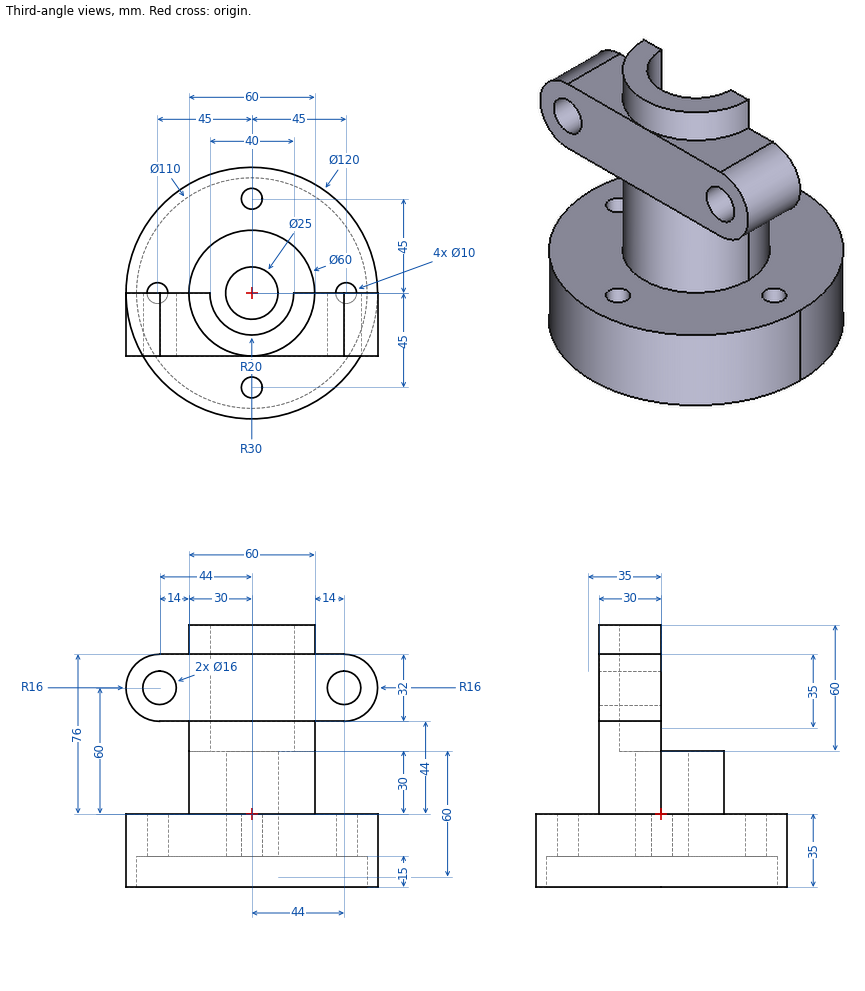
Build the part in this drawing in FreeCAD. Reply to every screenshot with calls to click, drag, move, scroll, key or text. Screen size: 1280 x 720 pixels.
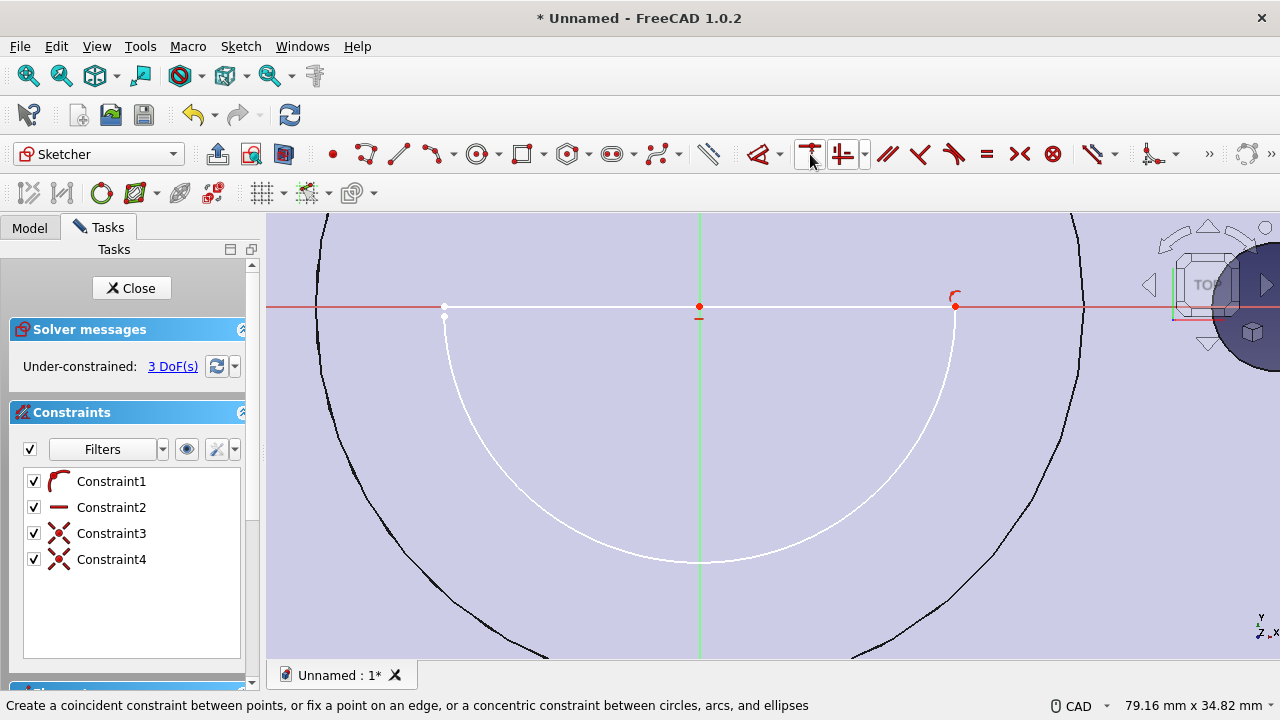
click(758, 154)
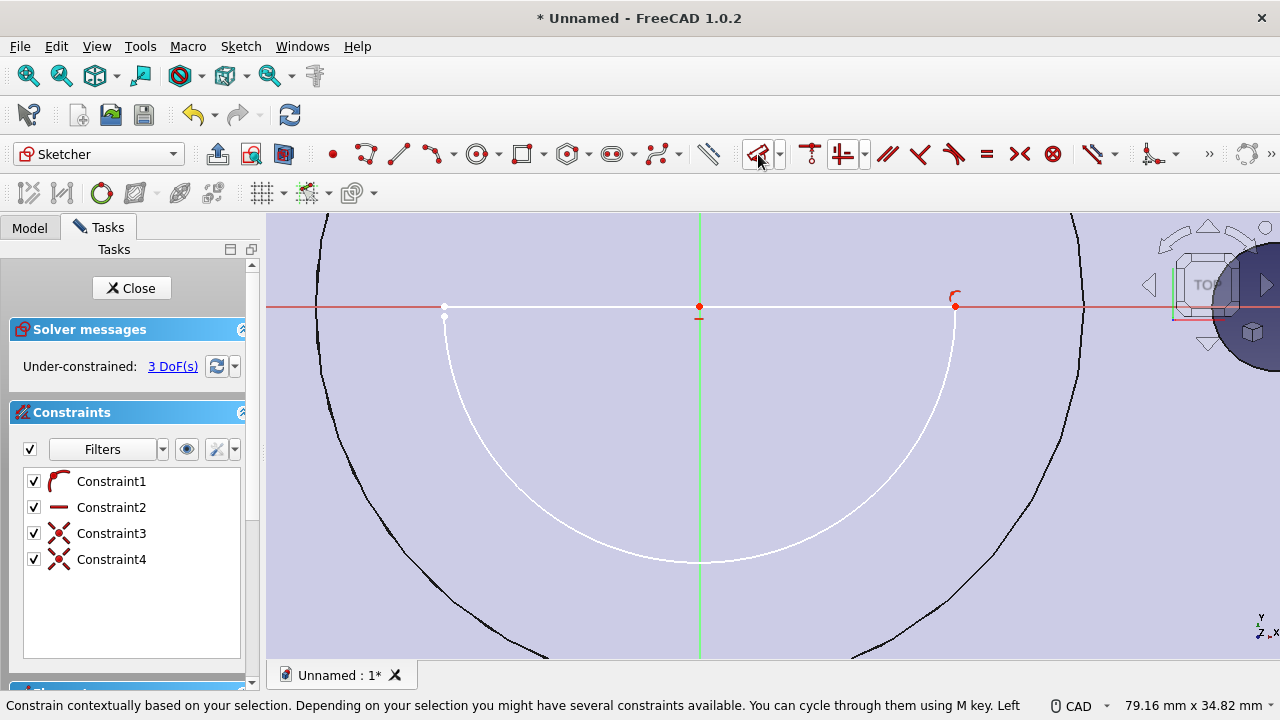
click(555, 518)
click(537, 544)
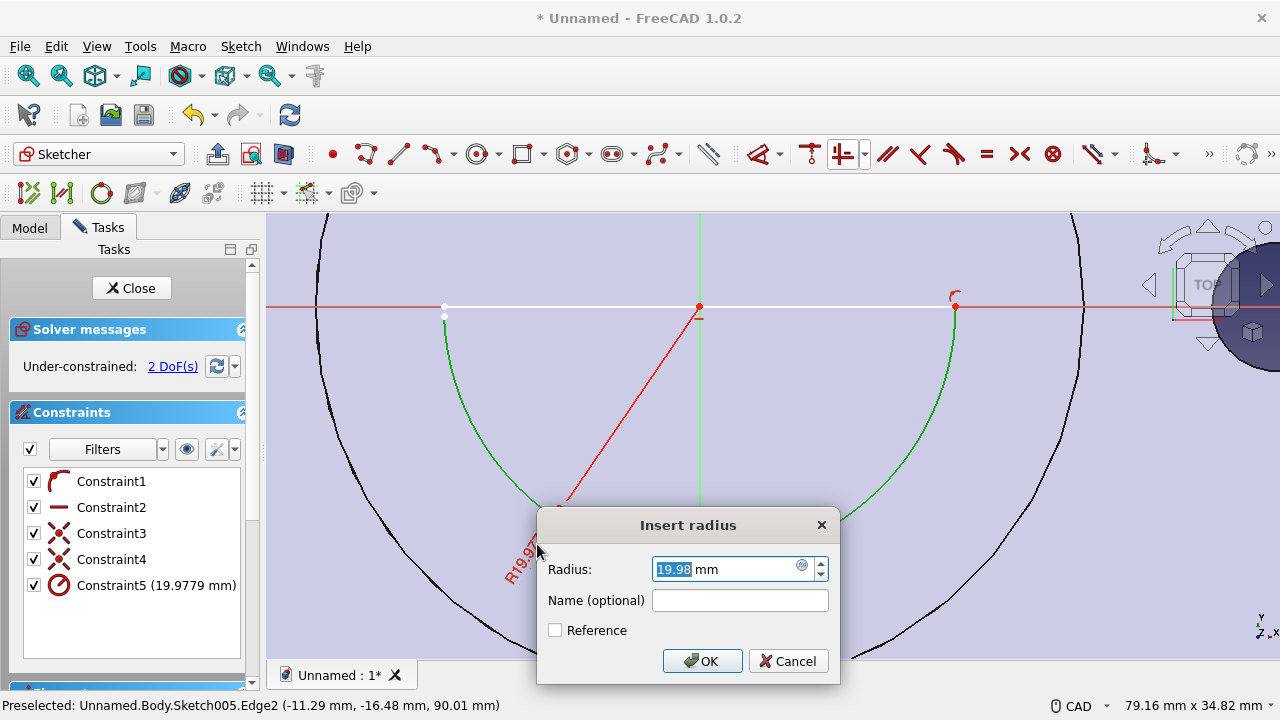
text(20)
key(Return)
key(Escape)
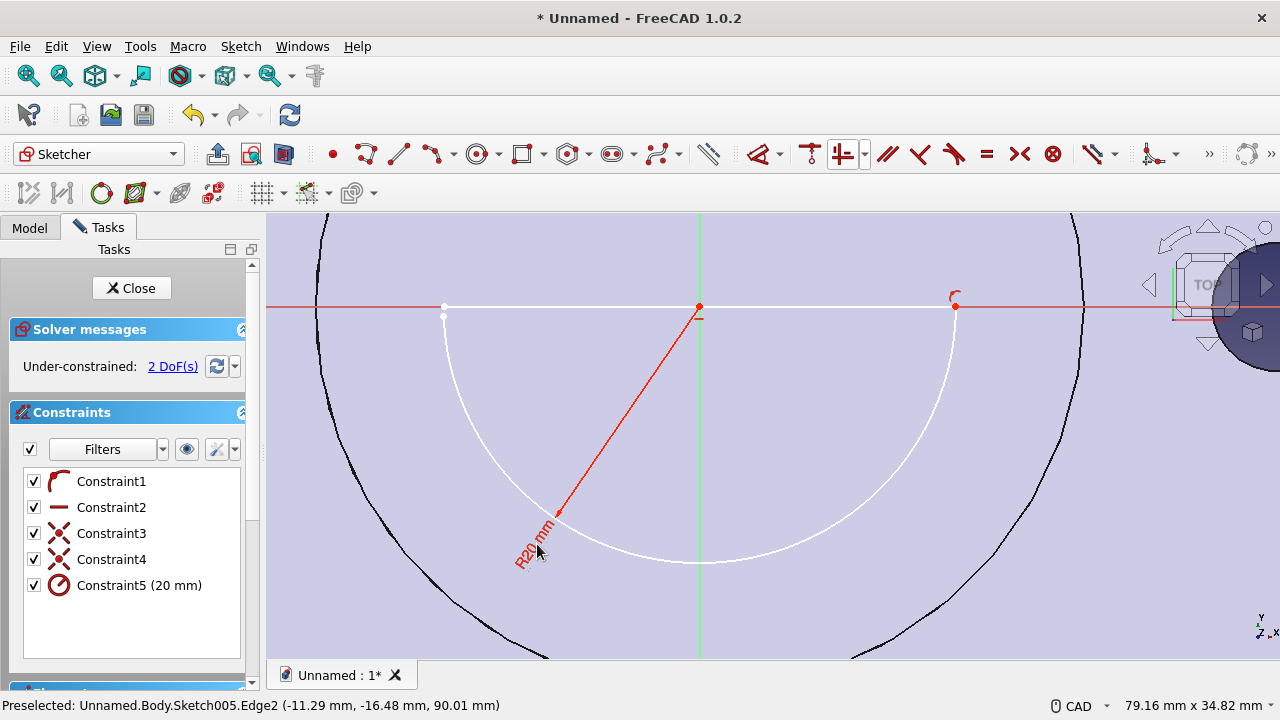
click(444, 317)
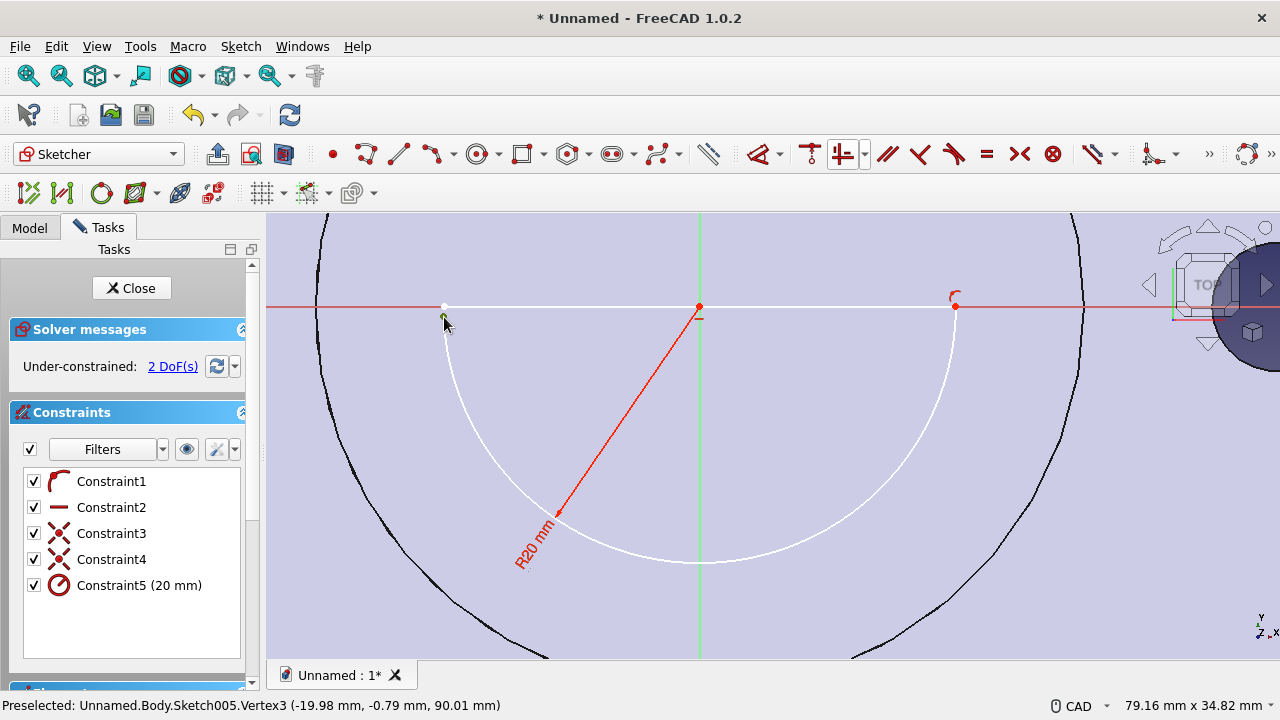
click(353, 307)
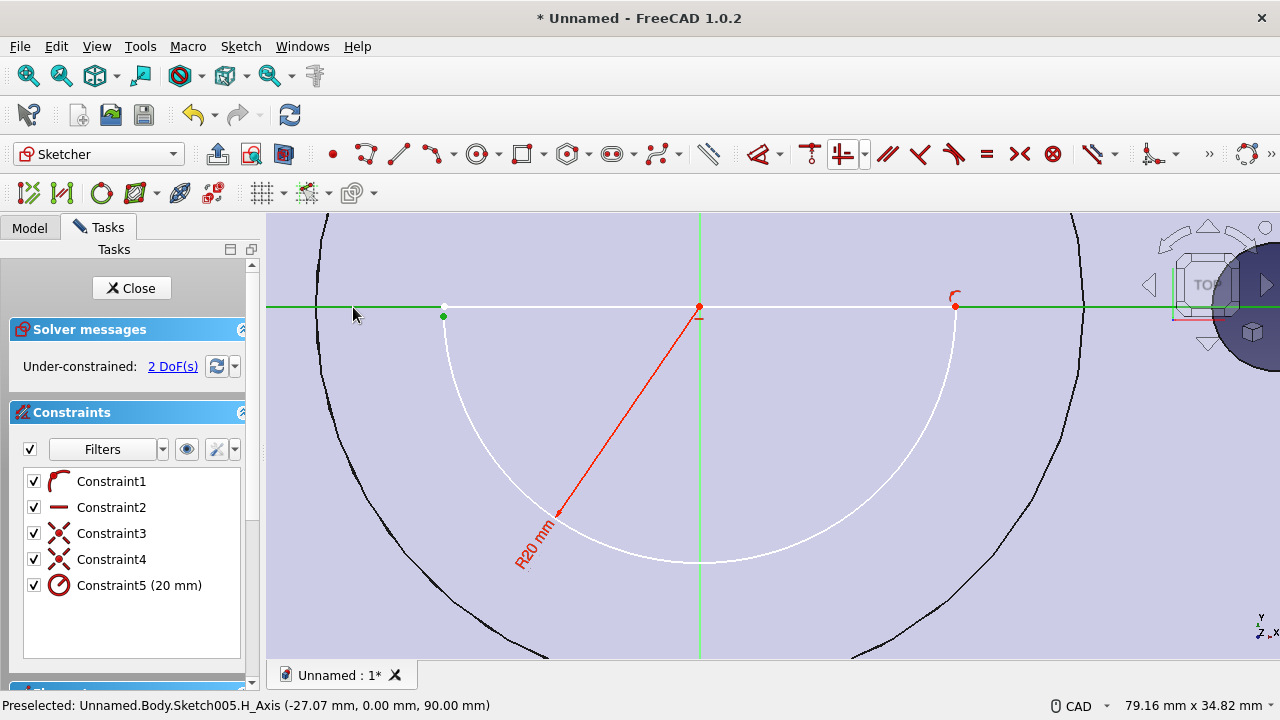
click(810, 154)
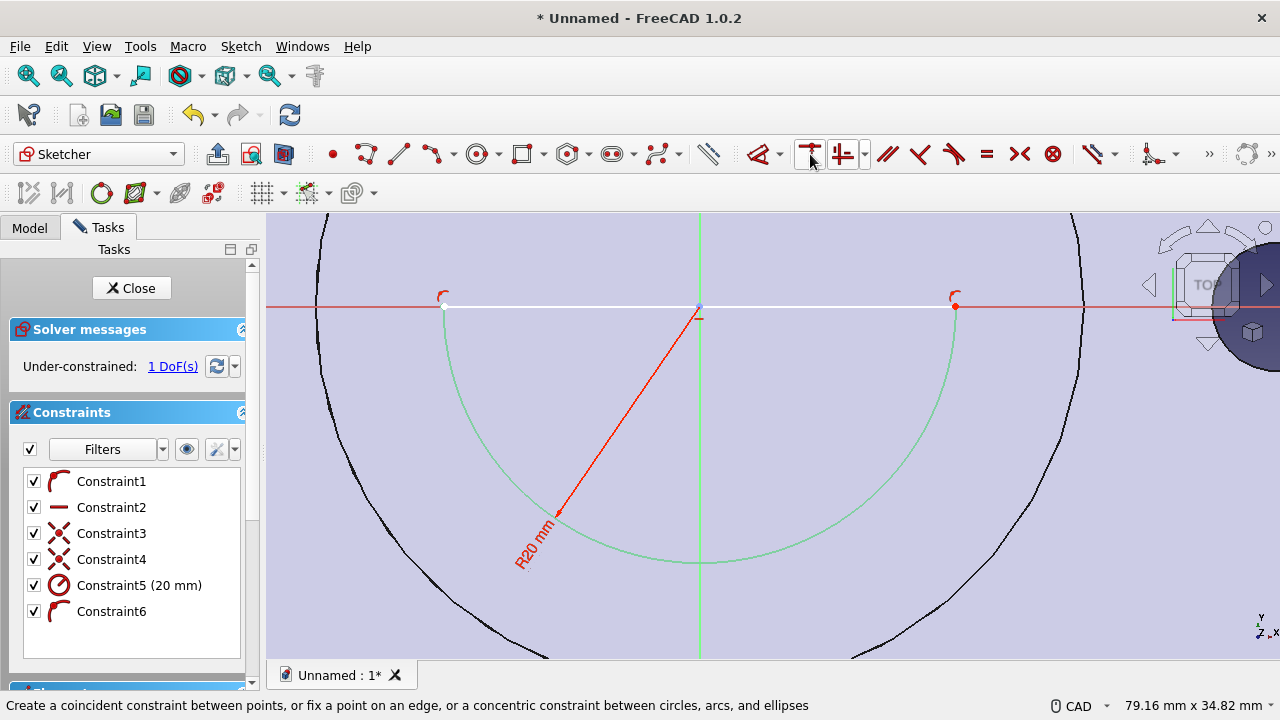
click(758, 154)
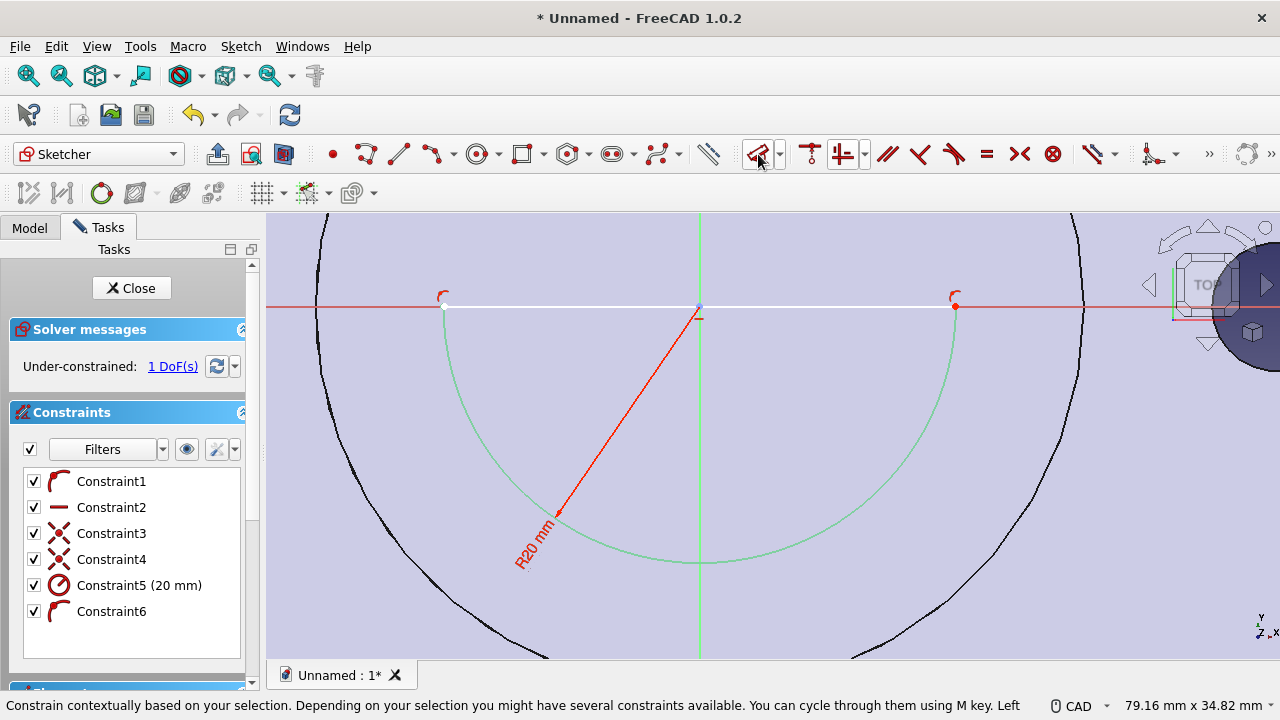
click(802, 307)
click(582, 273)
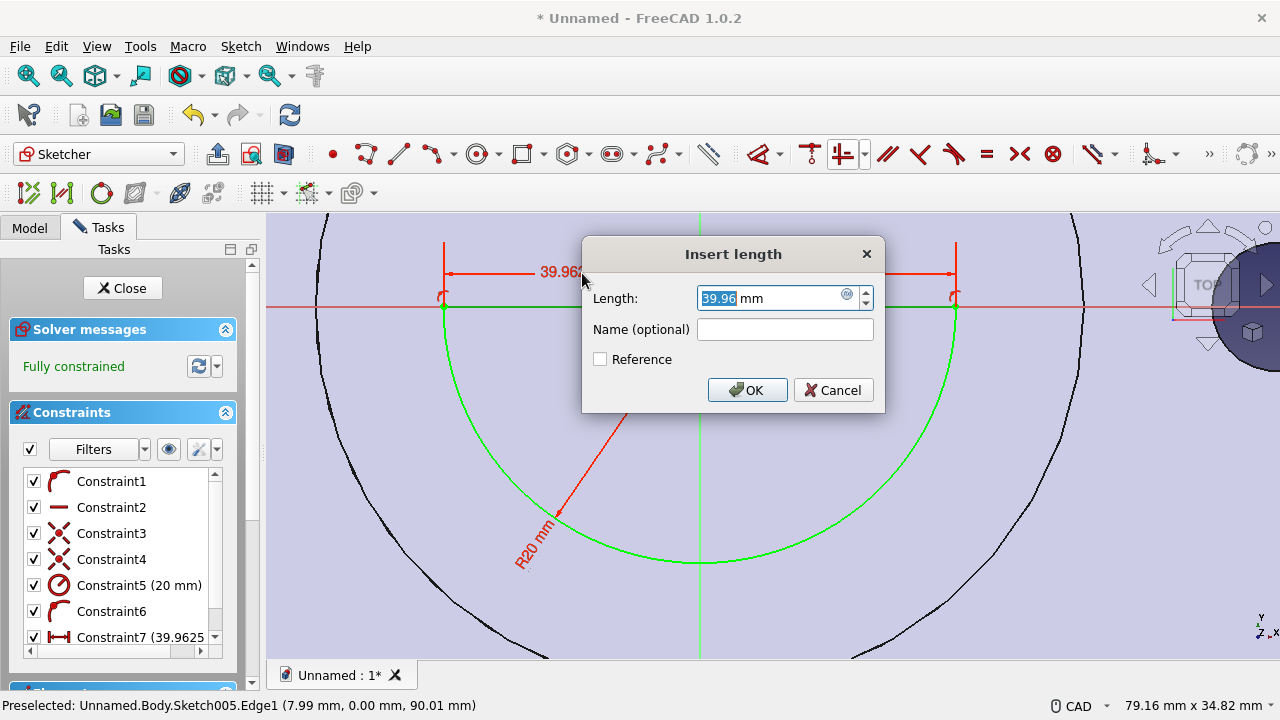
text(40)
key(Return)
key(Escape)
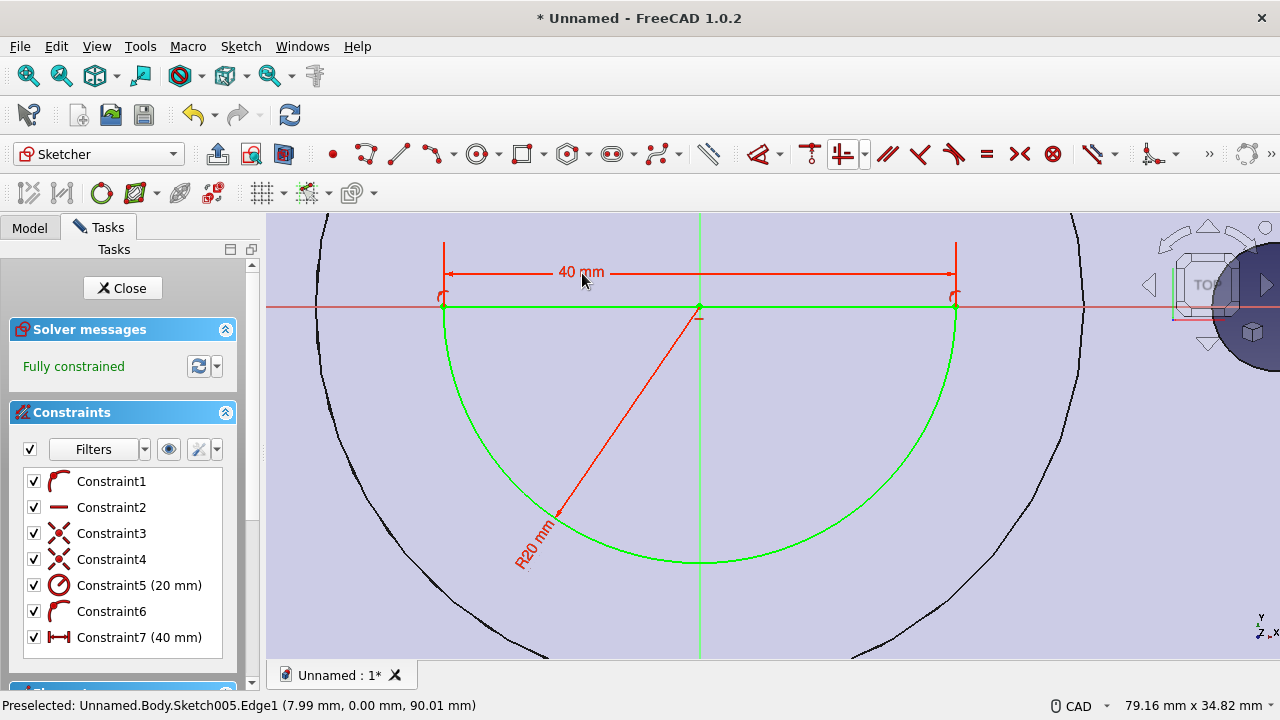
click(123, 288)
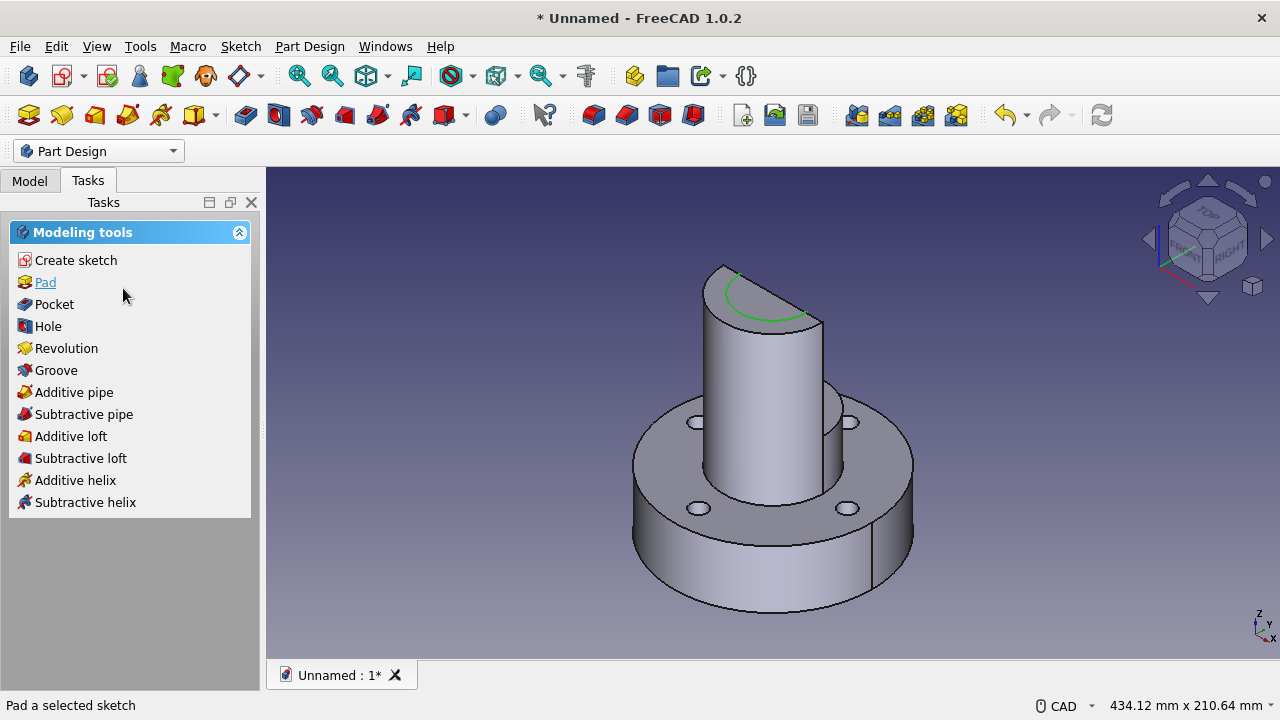
click(246, 116)